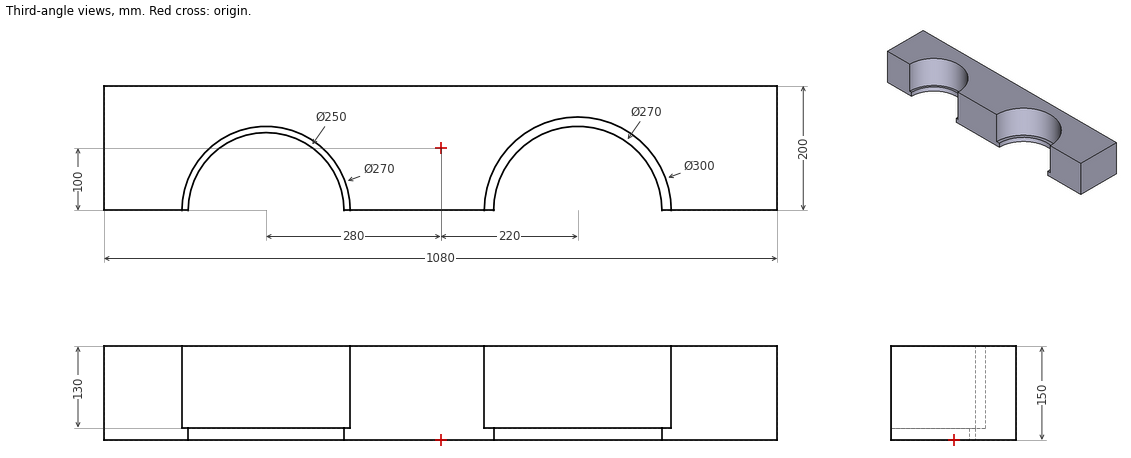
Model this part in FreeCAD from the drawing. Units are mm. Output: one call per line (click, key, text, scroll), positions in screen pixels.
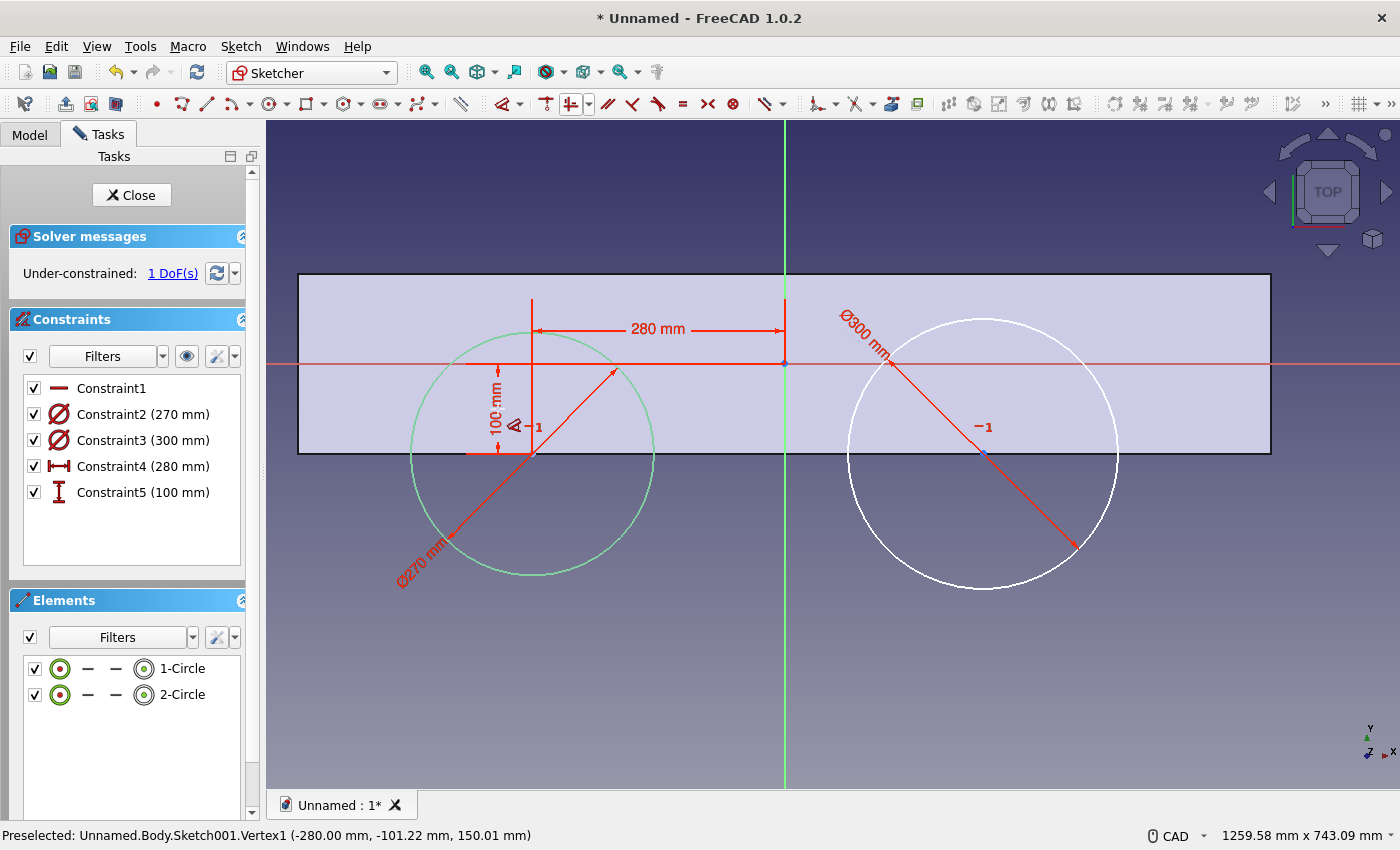
click(983, 454)
click(884, 488)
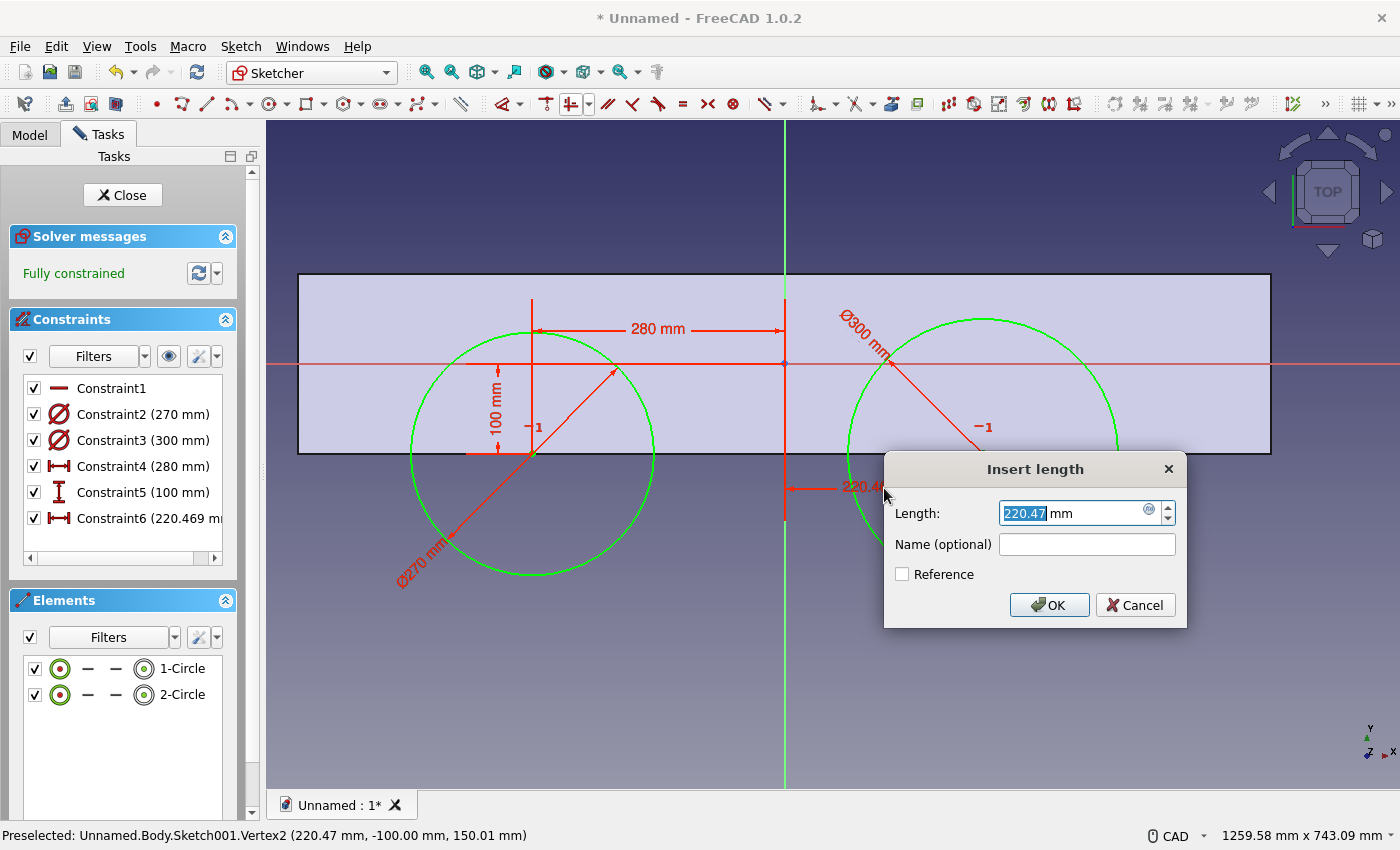
text(220)
key(Return)
key(Escape)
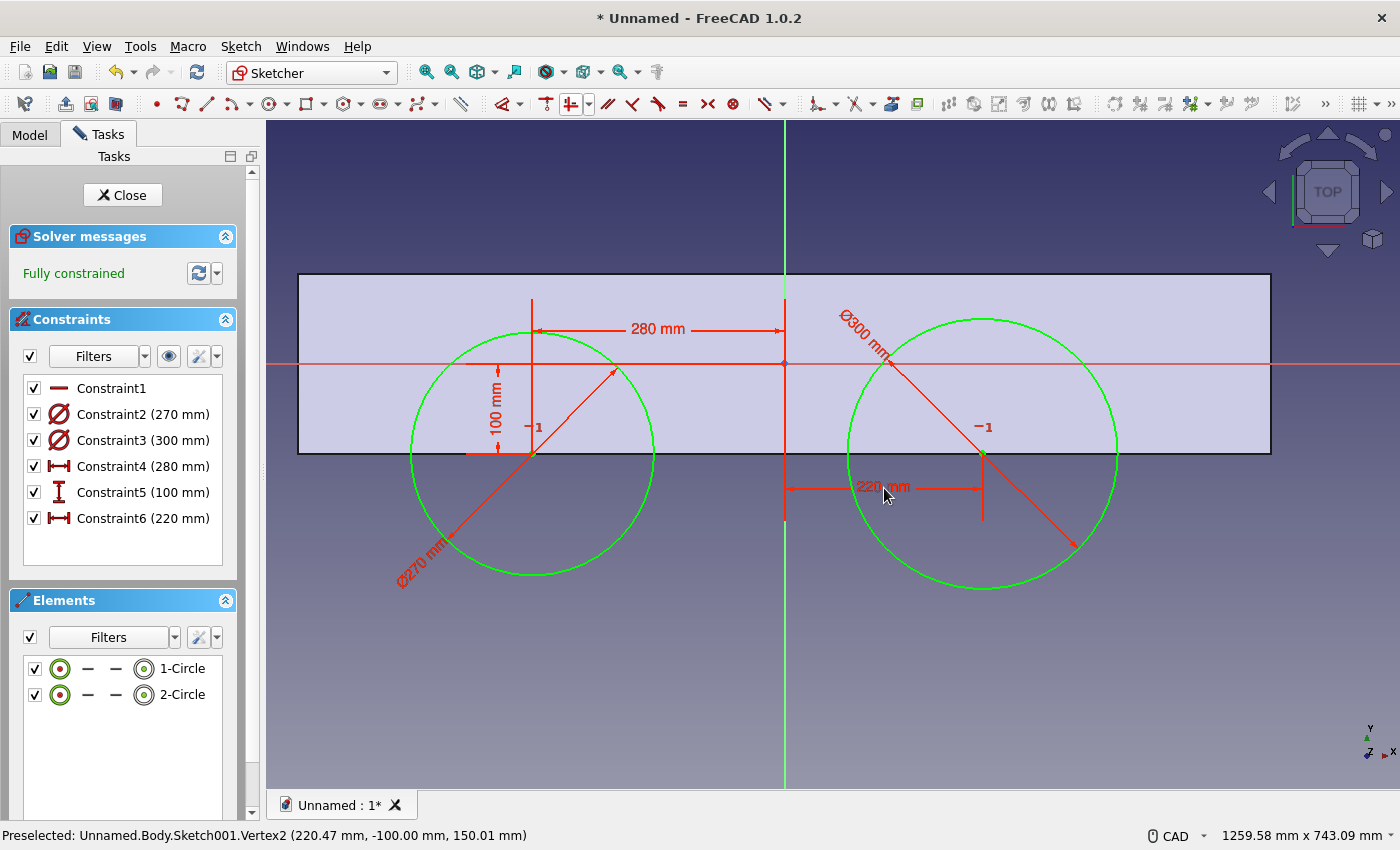
click(123, 195)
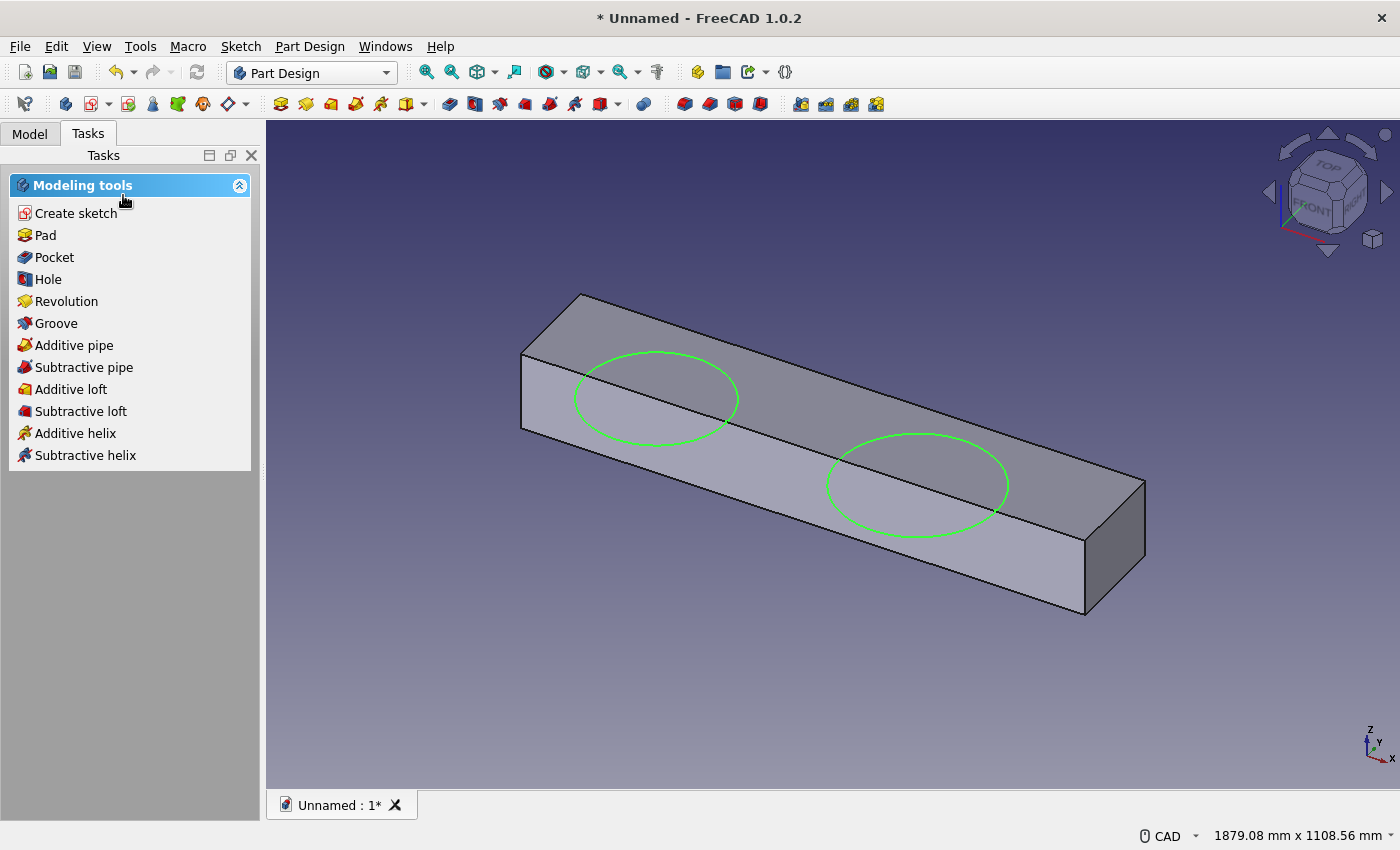
click(450, 104)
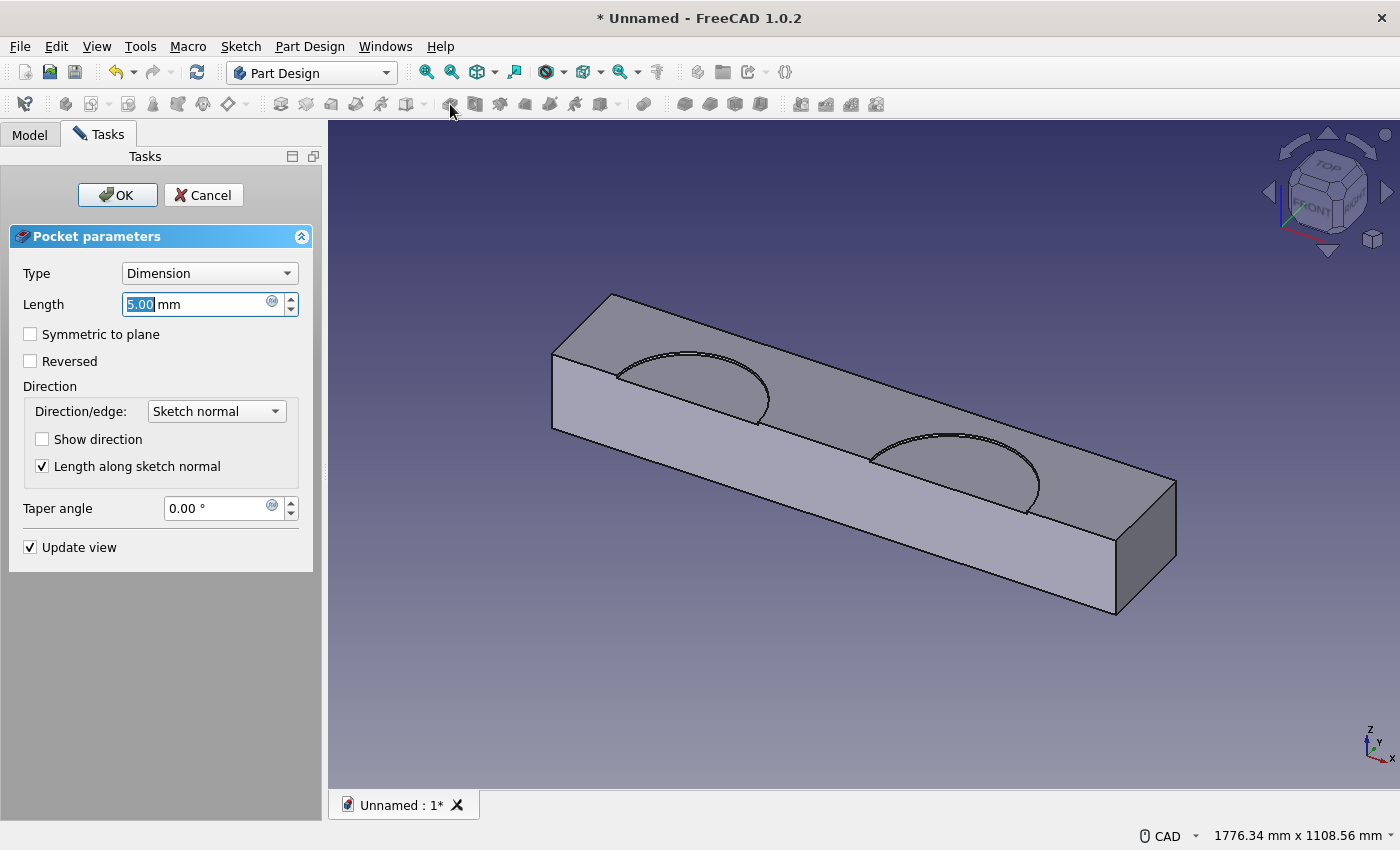
text(130)
key(Tab)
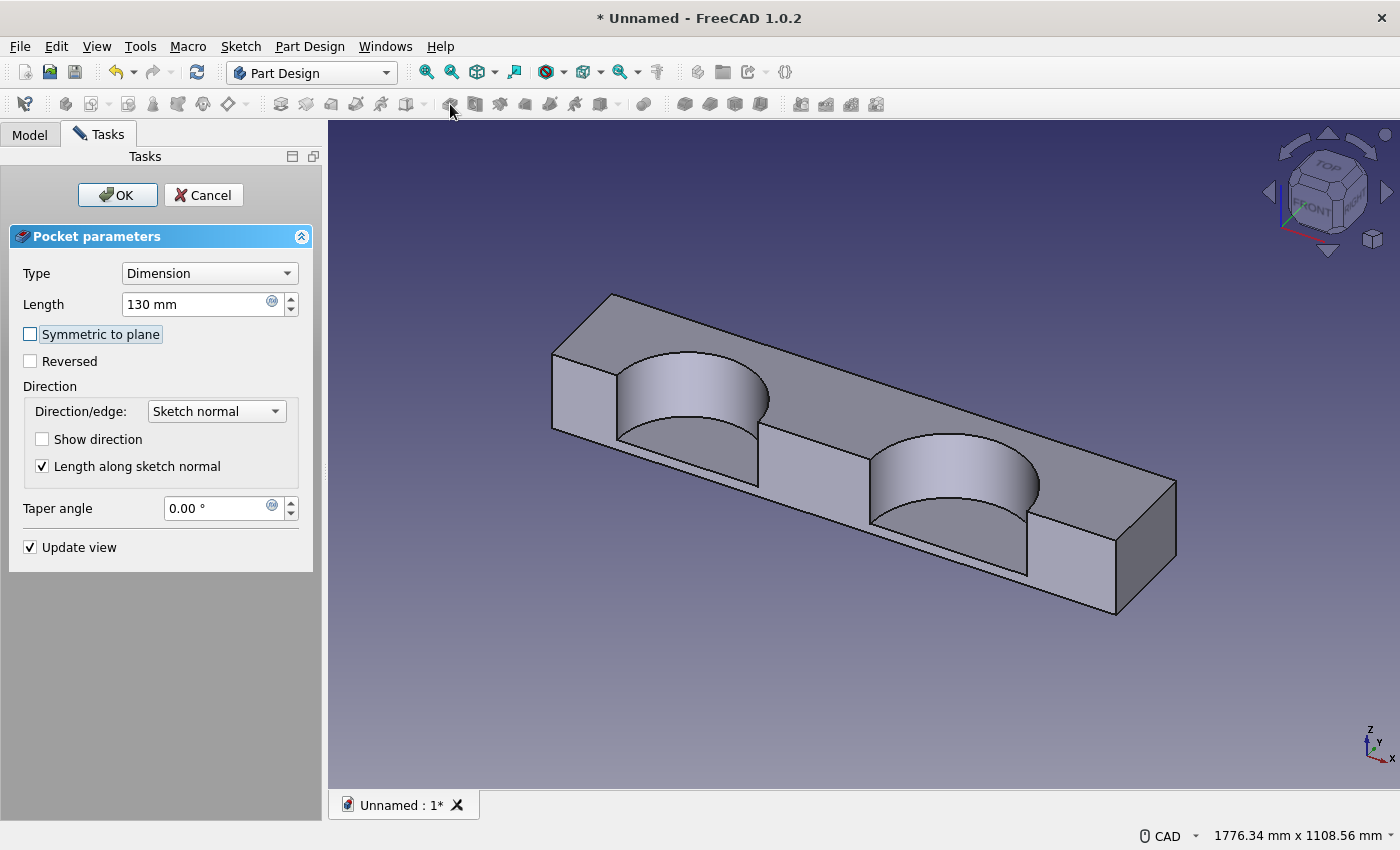
click(118, 195)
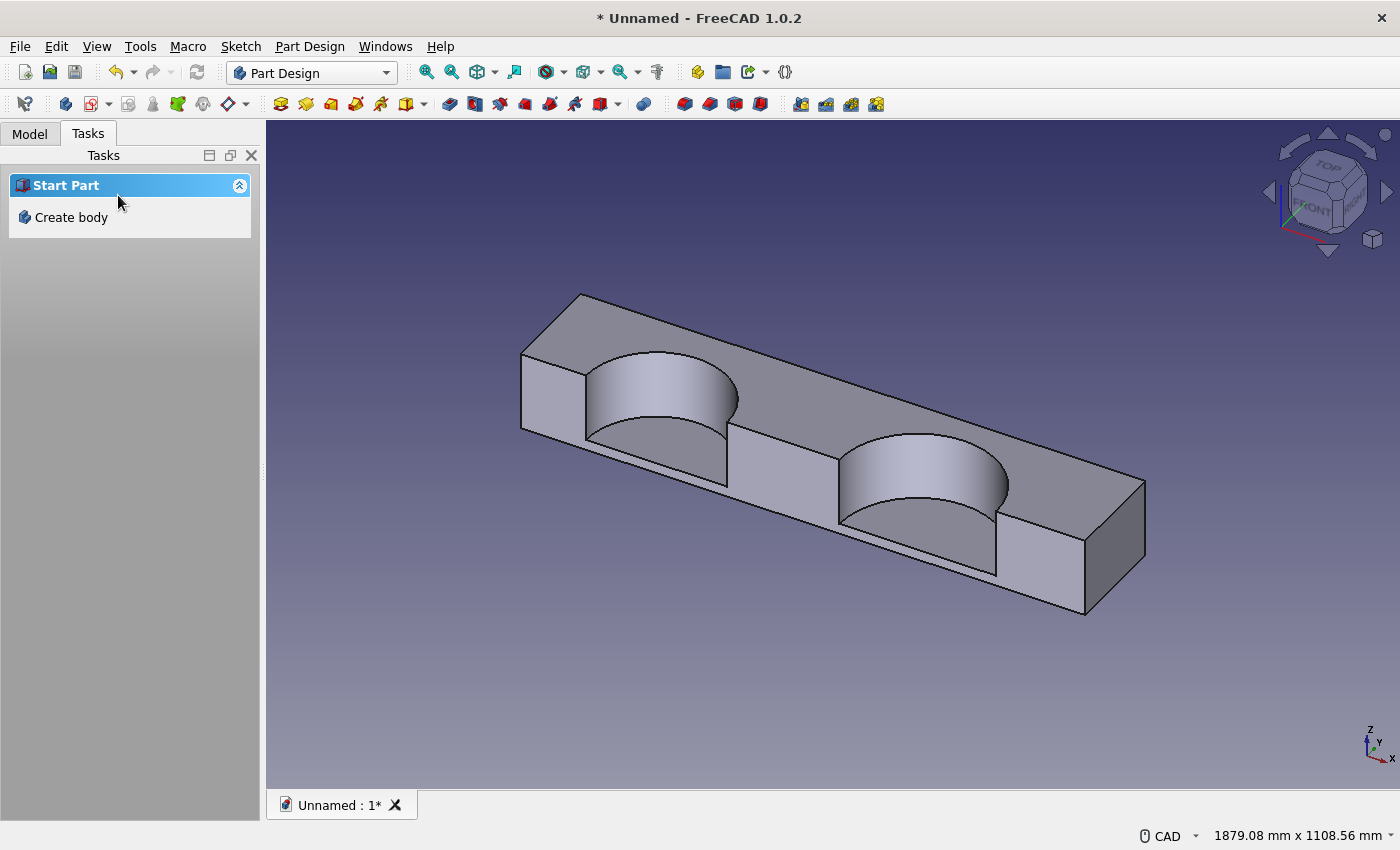
click(833, 416)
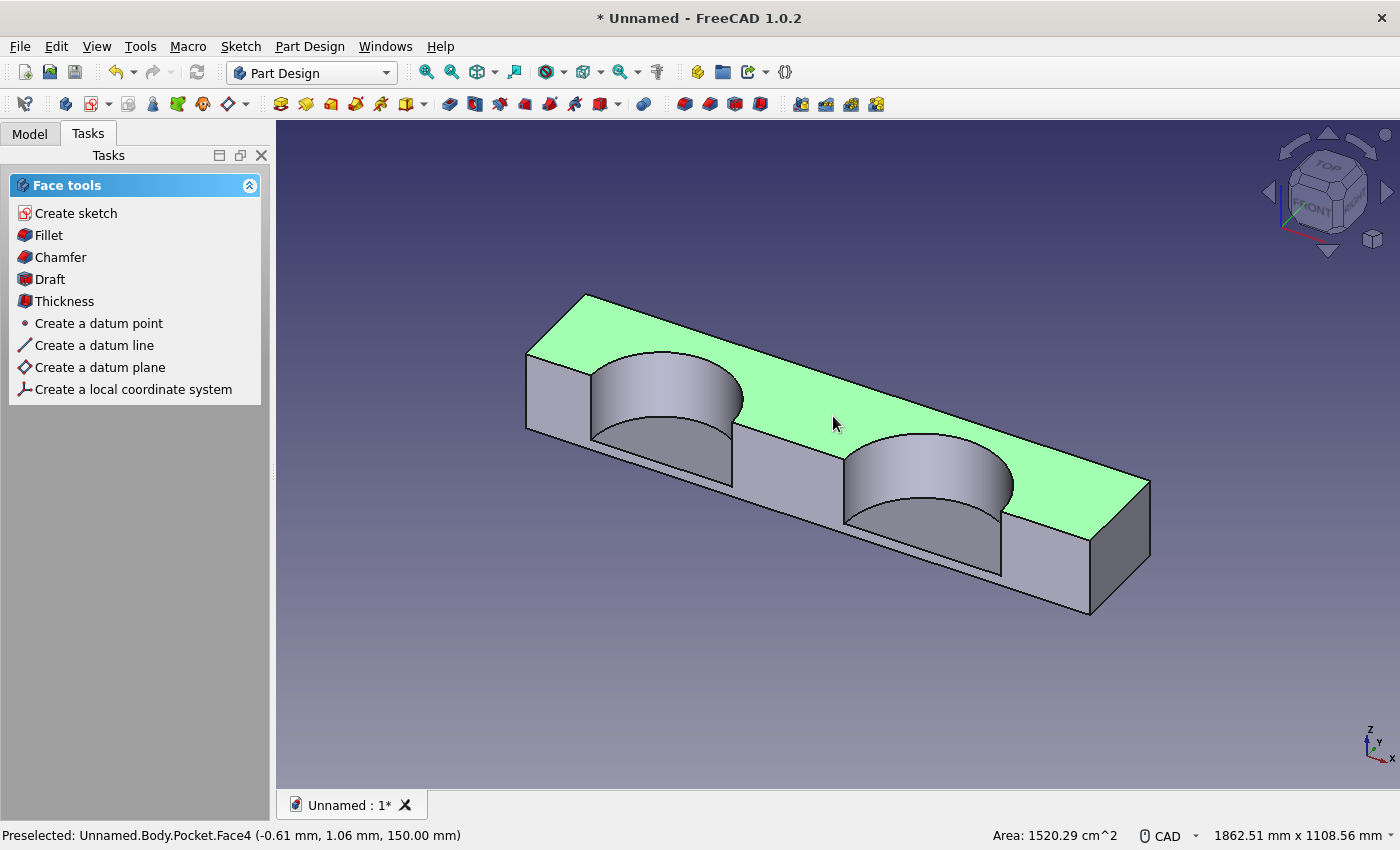
click(90, 104)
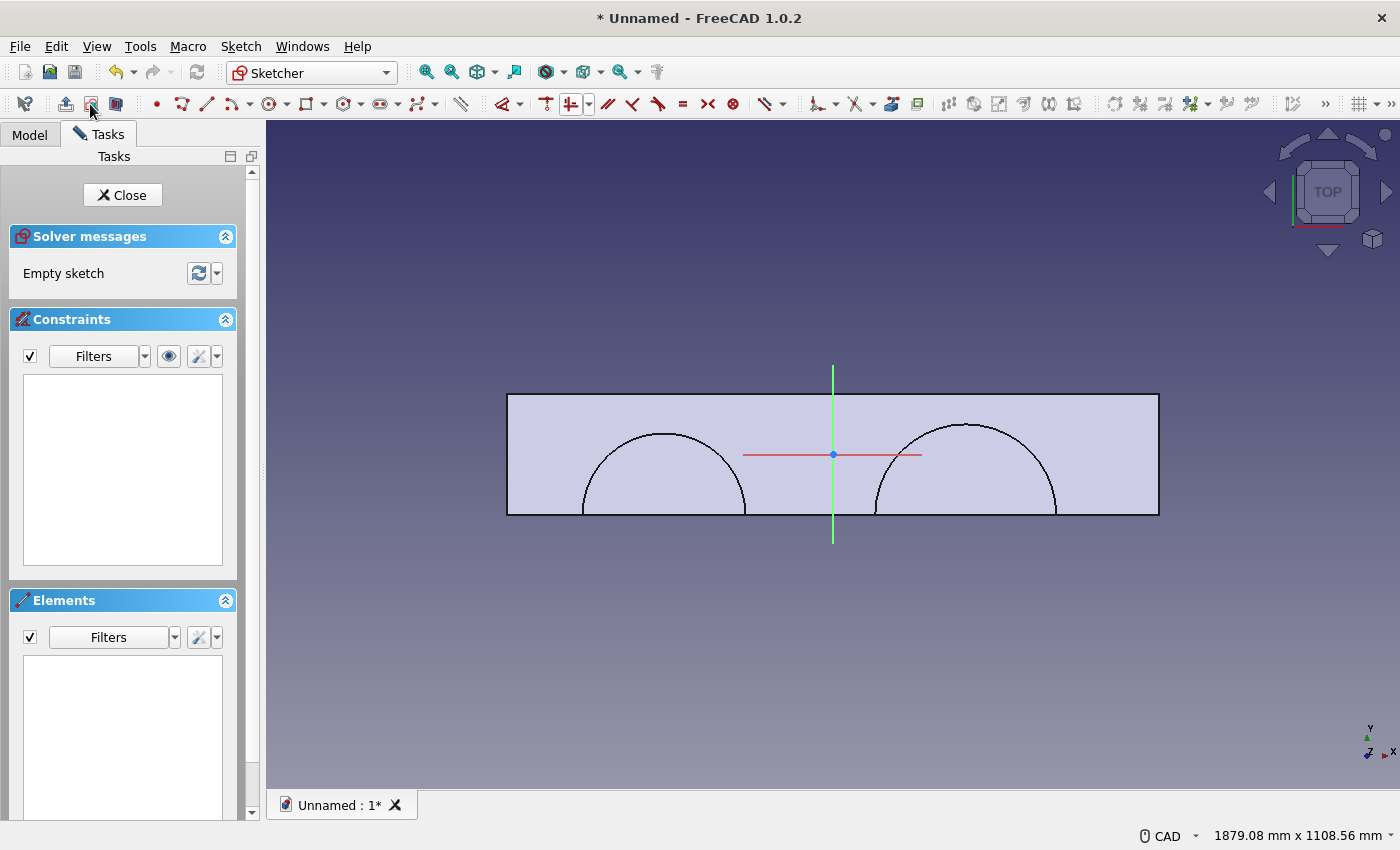
scroll(927, 638, up, 2)